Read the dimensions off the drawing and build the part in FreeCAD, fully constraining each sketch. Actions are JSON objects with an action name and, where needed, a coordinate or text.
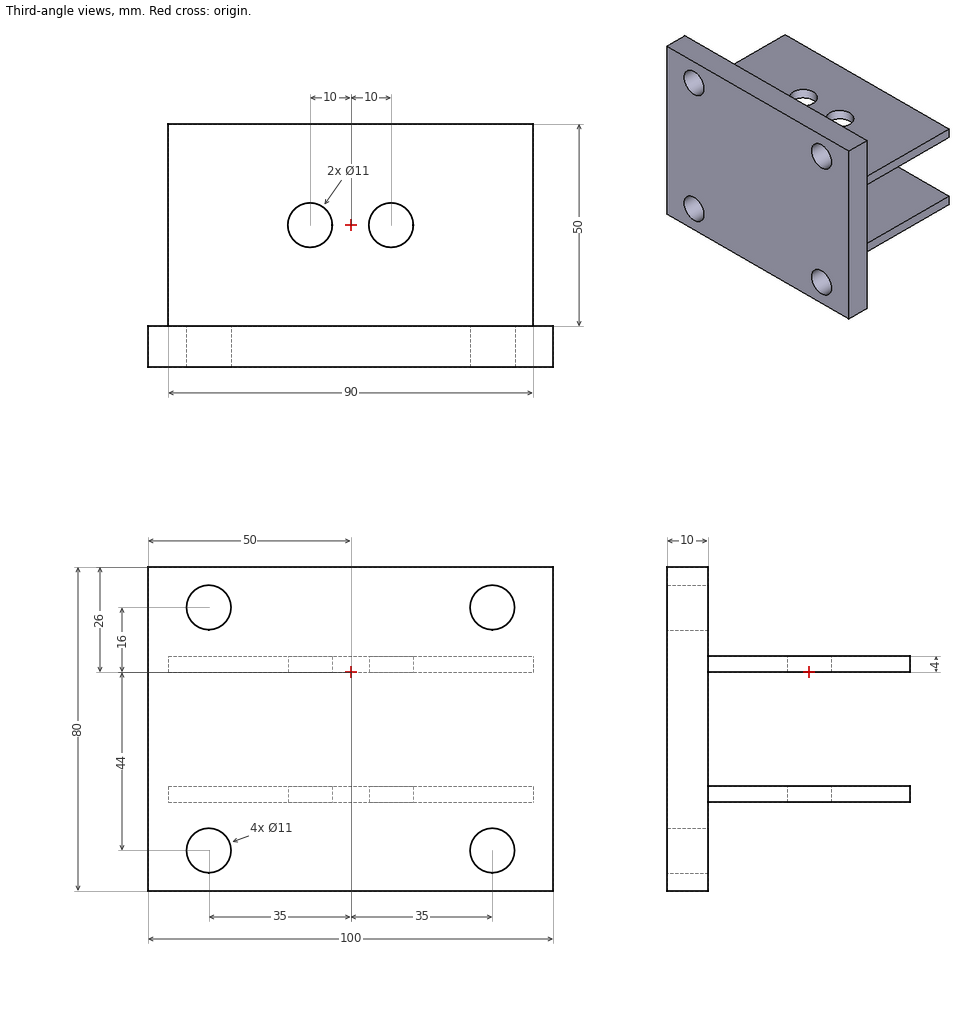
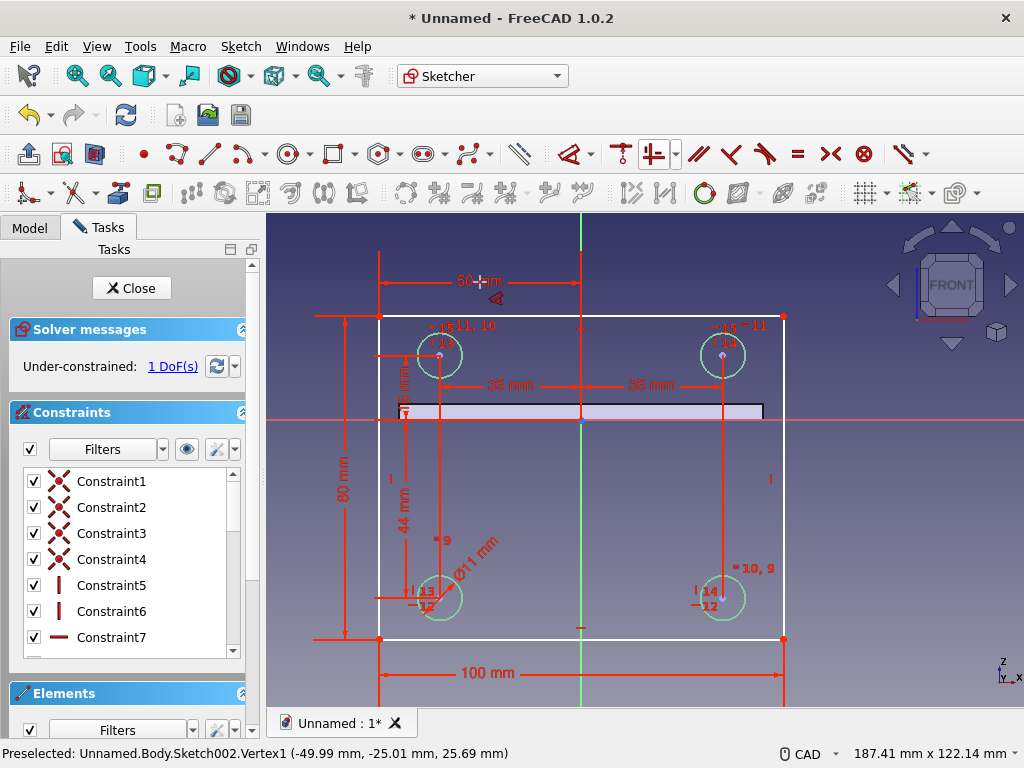
{"action": "left_click", "coordinate": [379, 316]}
{"action": "left_click", "coordinate": [345, 368]}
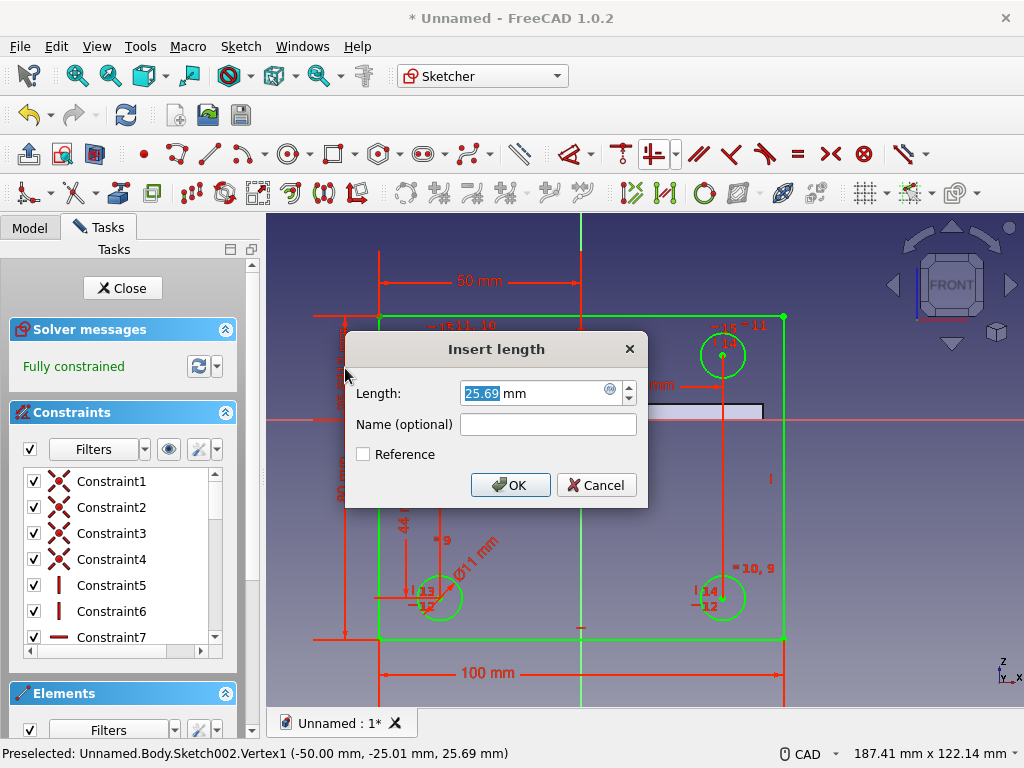
{"action": "type", "text": "26"}
{"action": "key", "text": "Return"}
{"action": "key", "text": "Escape"}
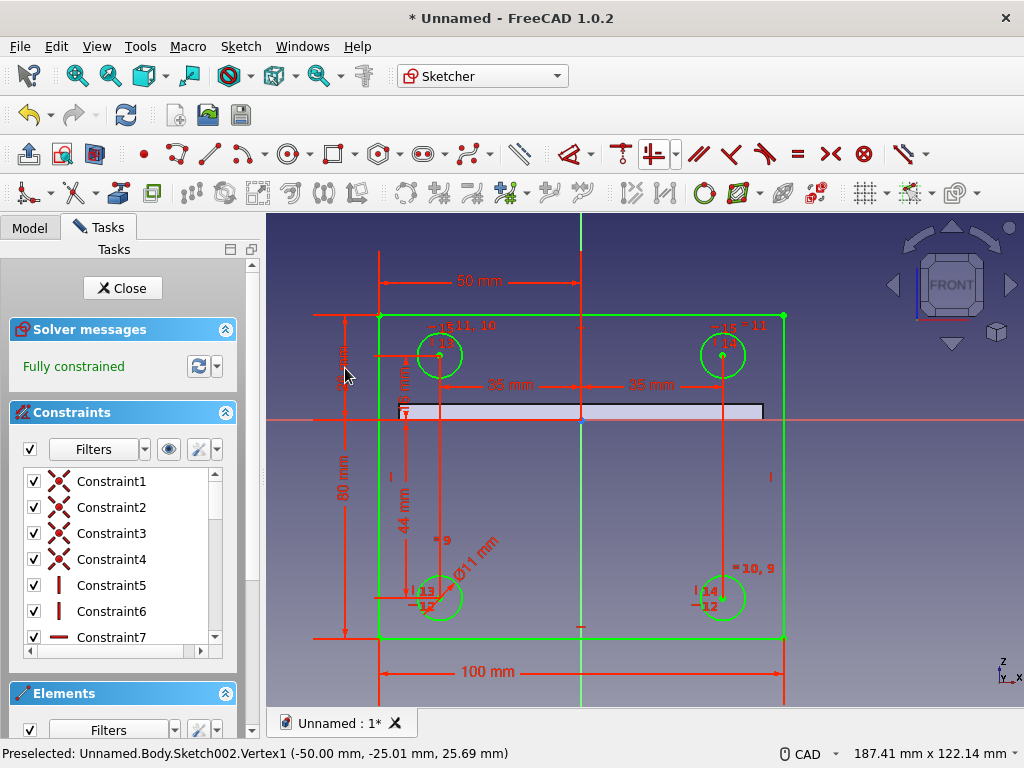
{"action": "left_click", "coordinate": [123, 288]}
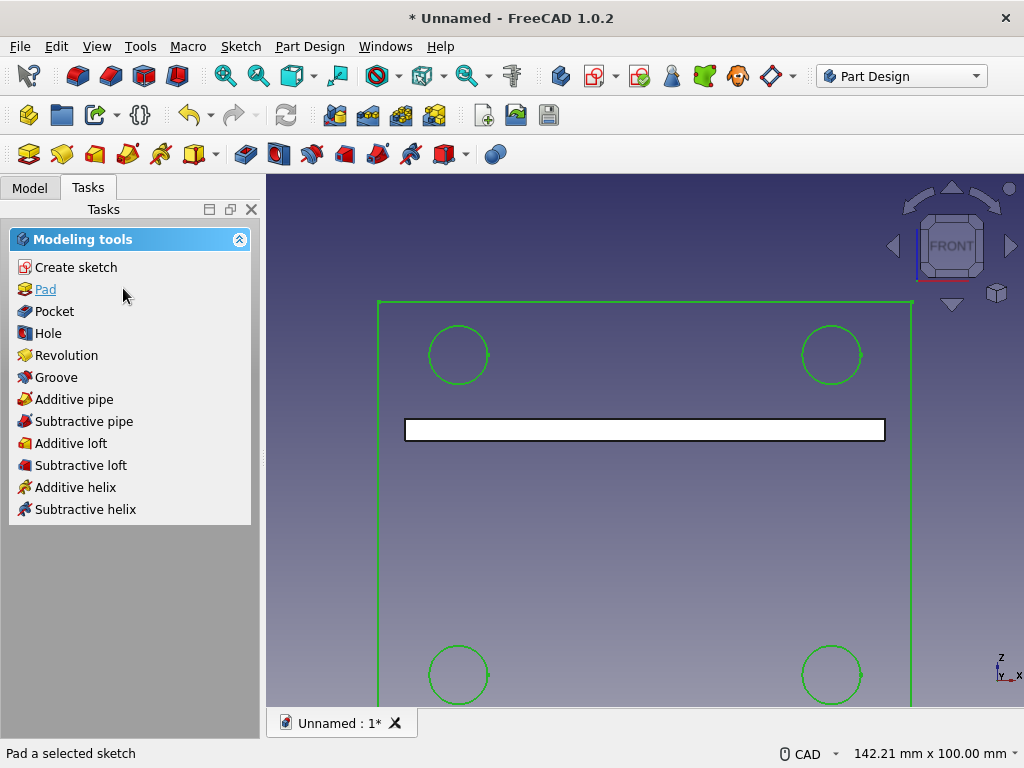
{"action": "left_click", "coordinate": [29, 154]}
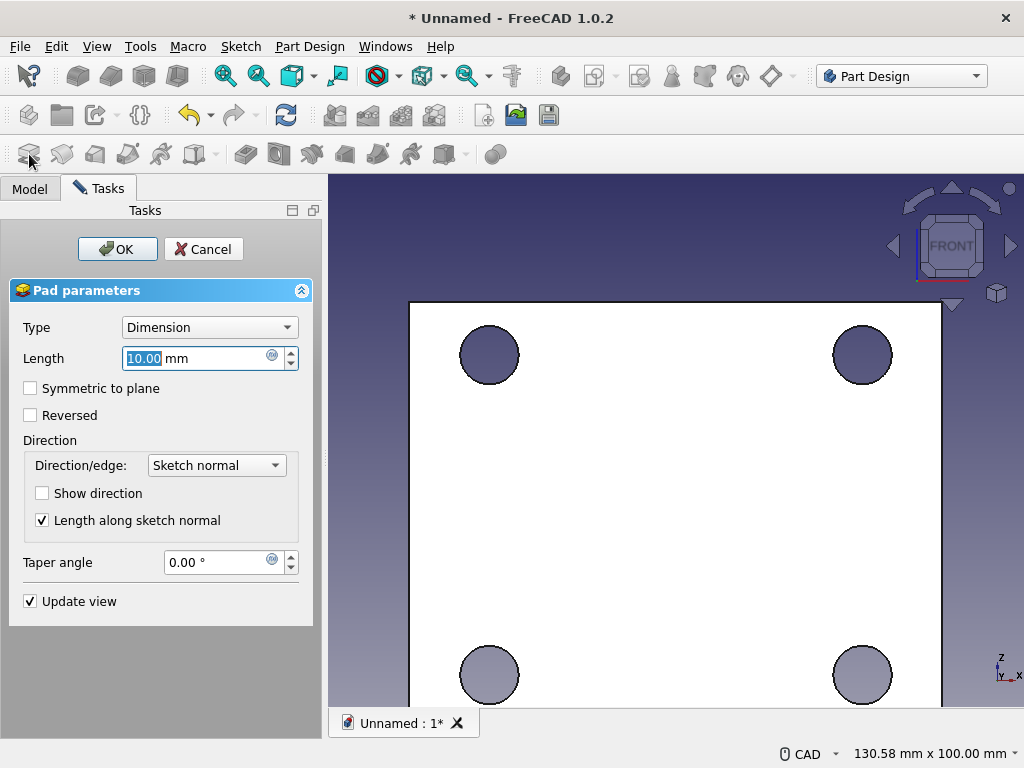
{"action": "type", "text": "10"}
{"action": "key", "text": "Tab"}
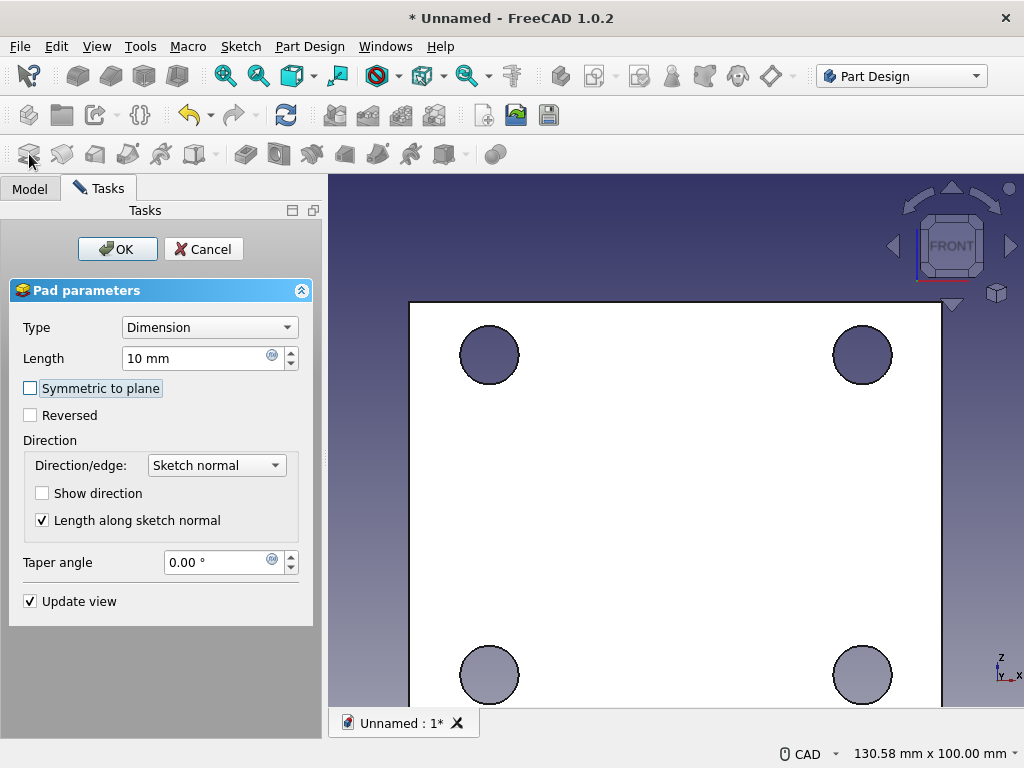
{"action": "left_click", "coordinate": [118, 249]}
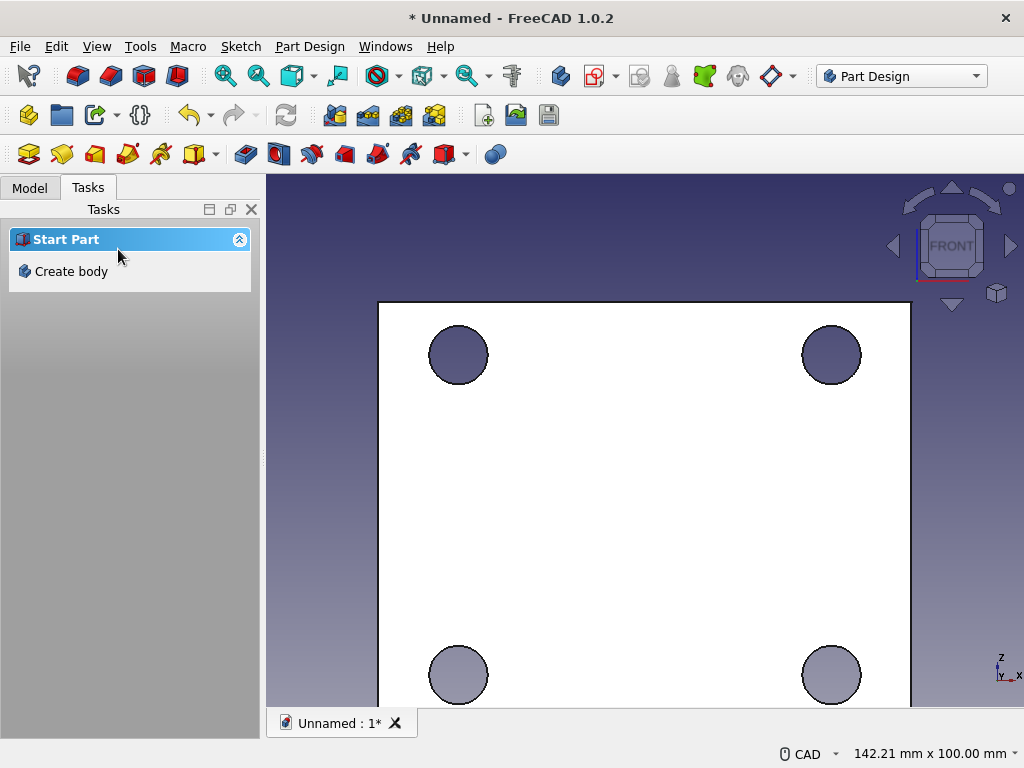
{"action": "key", "text": "v f"}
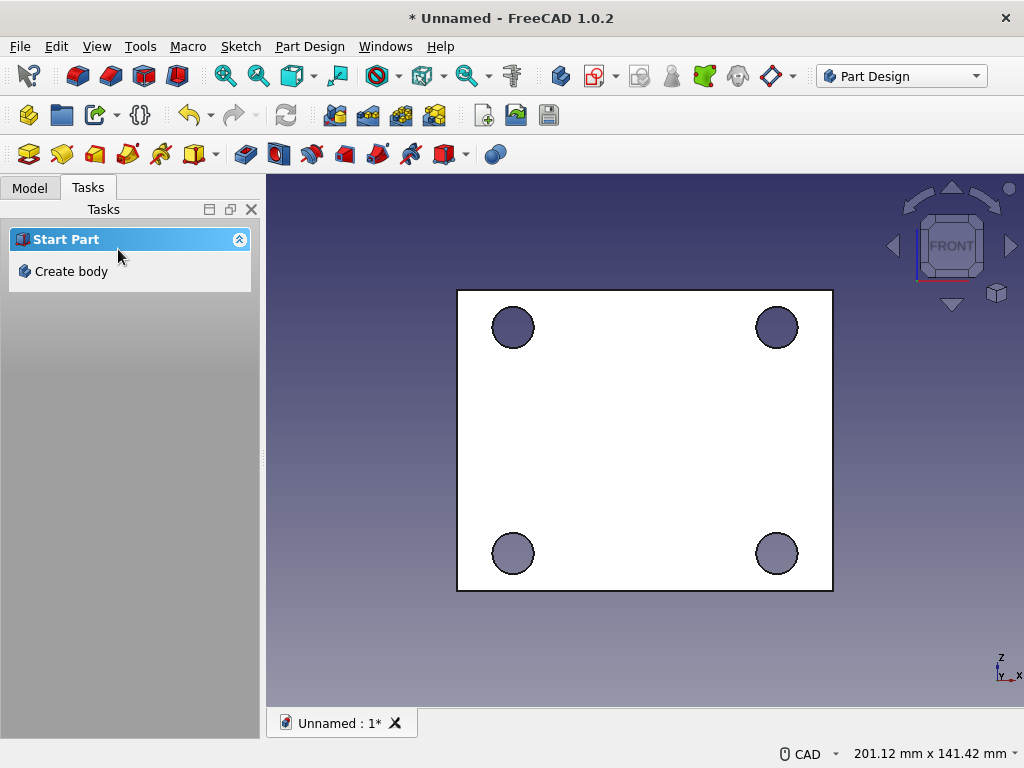
{"action": "left_click", "coordinate": [30, 188]}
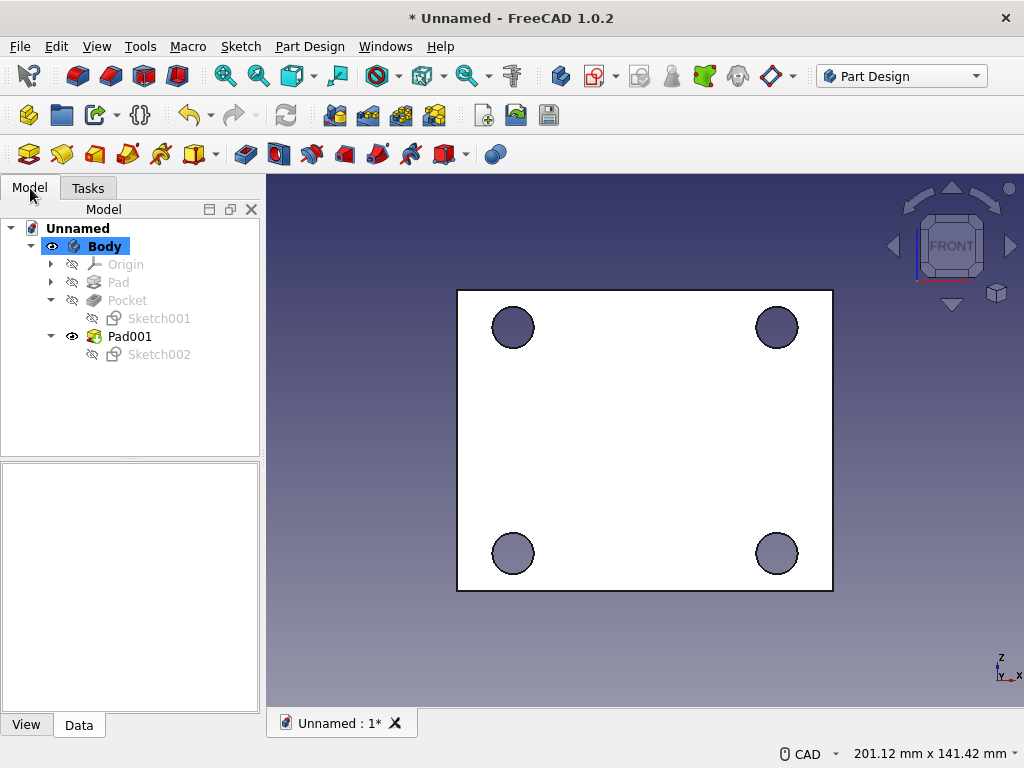
{"action": "left_click", "coordinate": [51, 264]}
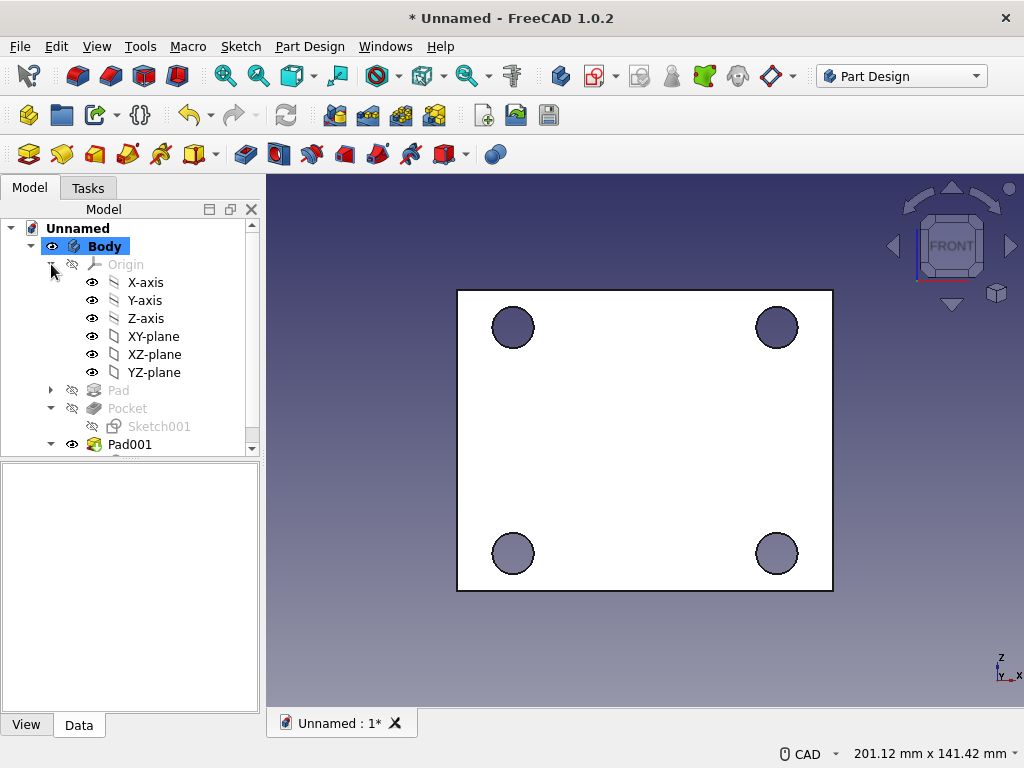
{"action": "left_click", "coordinate": [137, 336]}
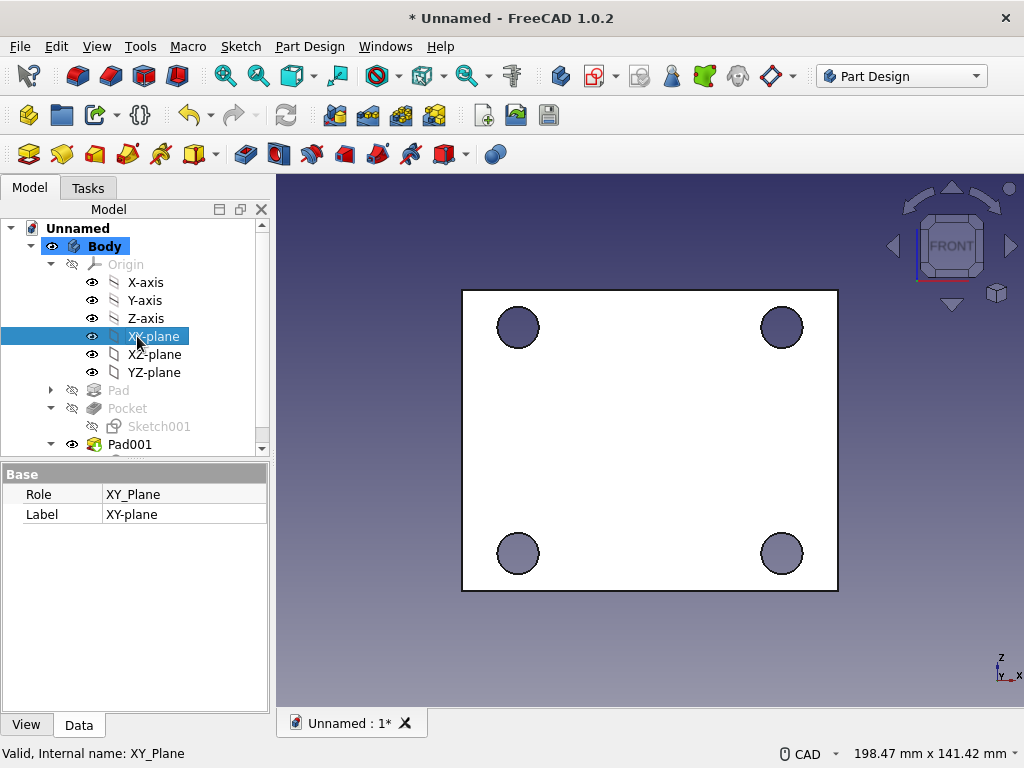
{"action": "left_click", "coordinate": [770, 76]}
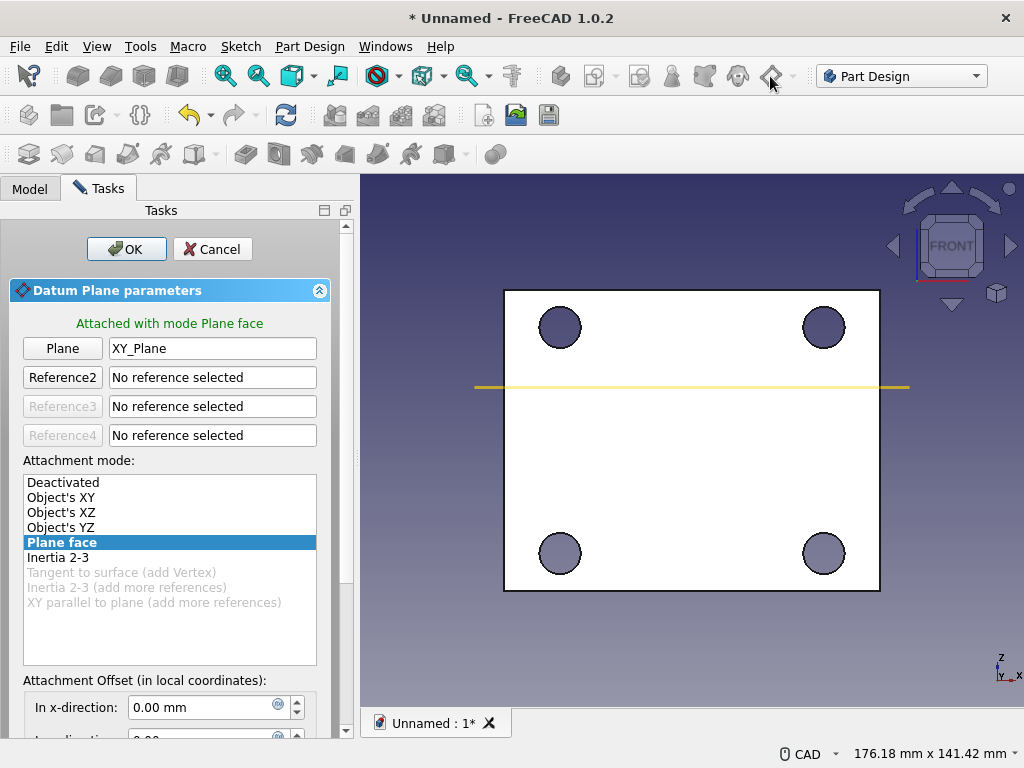
{"action": "scroll", "coordinate": [346, 479], "scroll_direction": "down", "scroll_amount": 2}